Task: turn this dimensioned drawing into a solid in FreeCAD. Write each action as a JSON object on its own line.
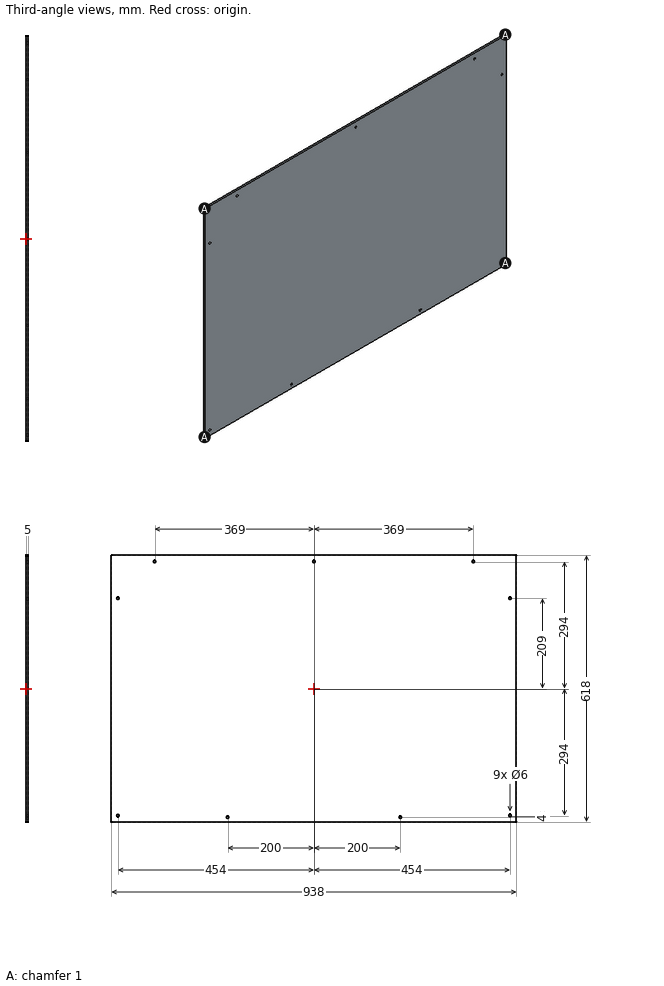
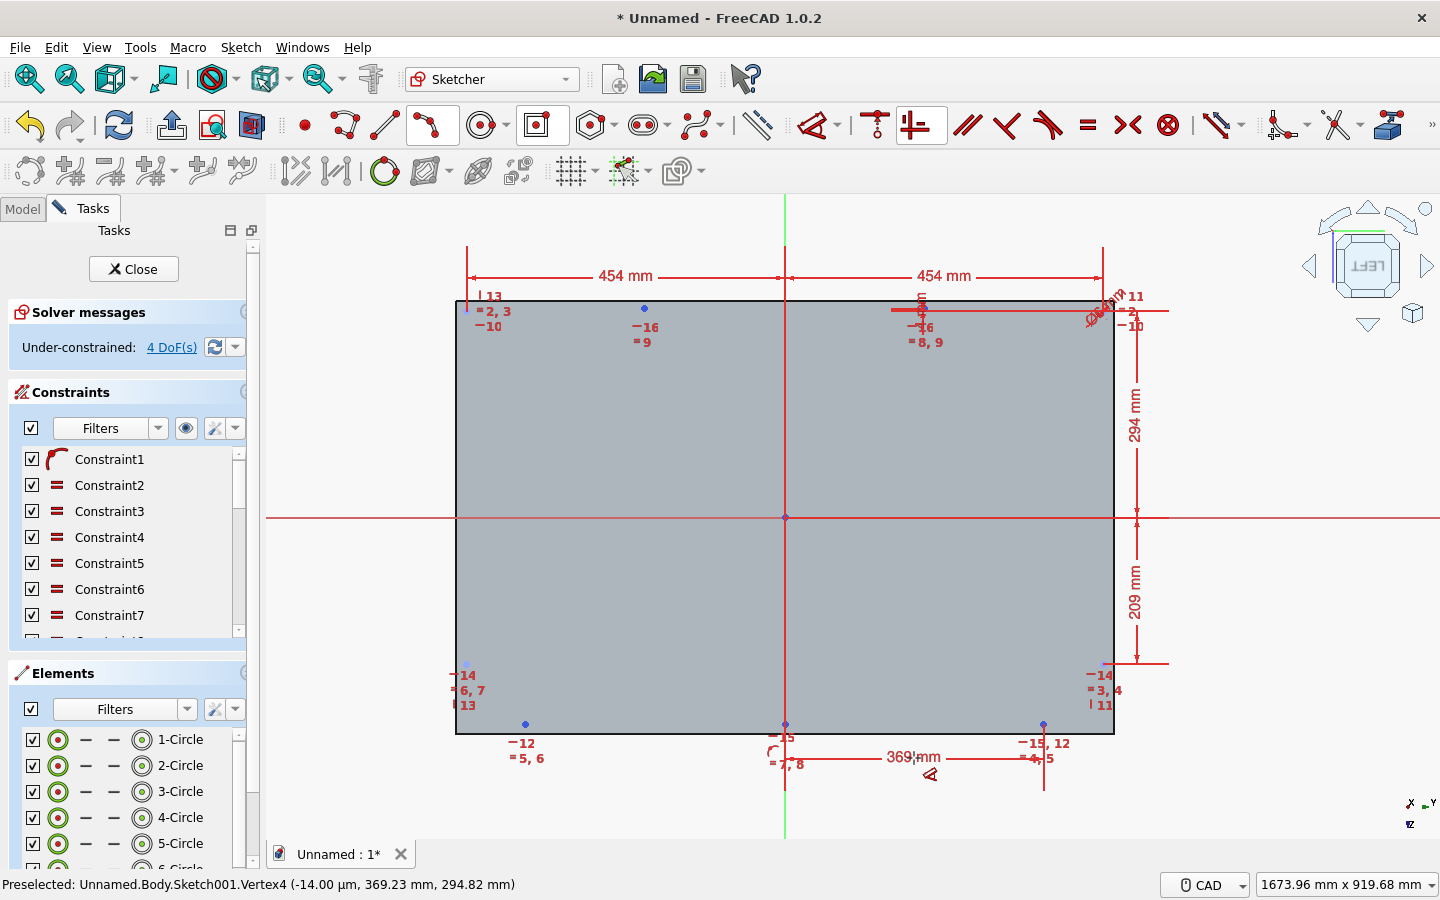
{"action": "left_click", "coordinate": [1044, 724]}
{"action": "left_click", "coordinate": [1078, 621]}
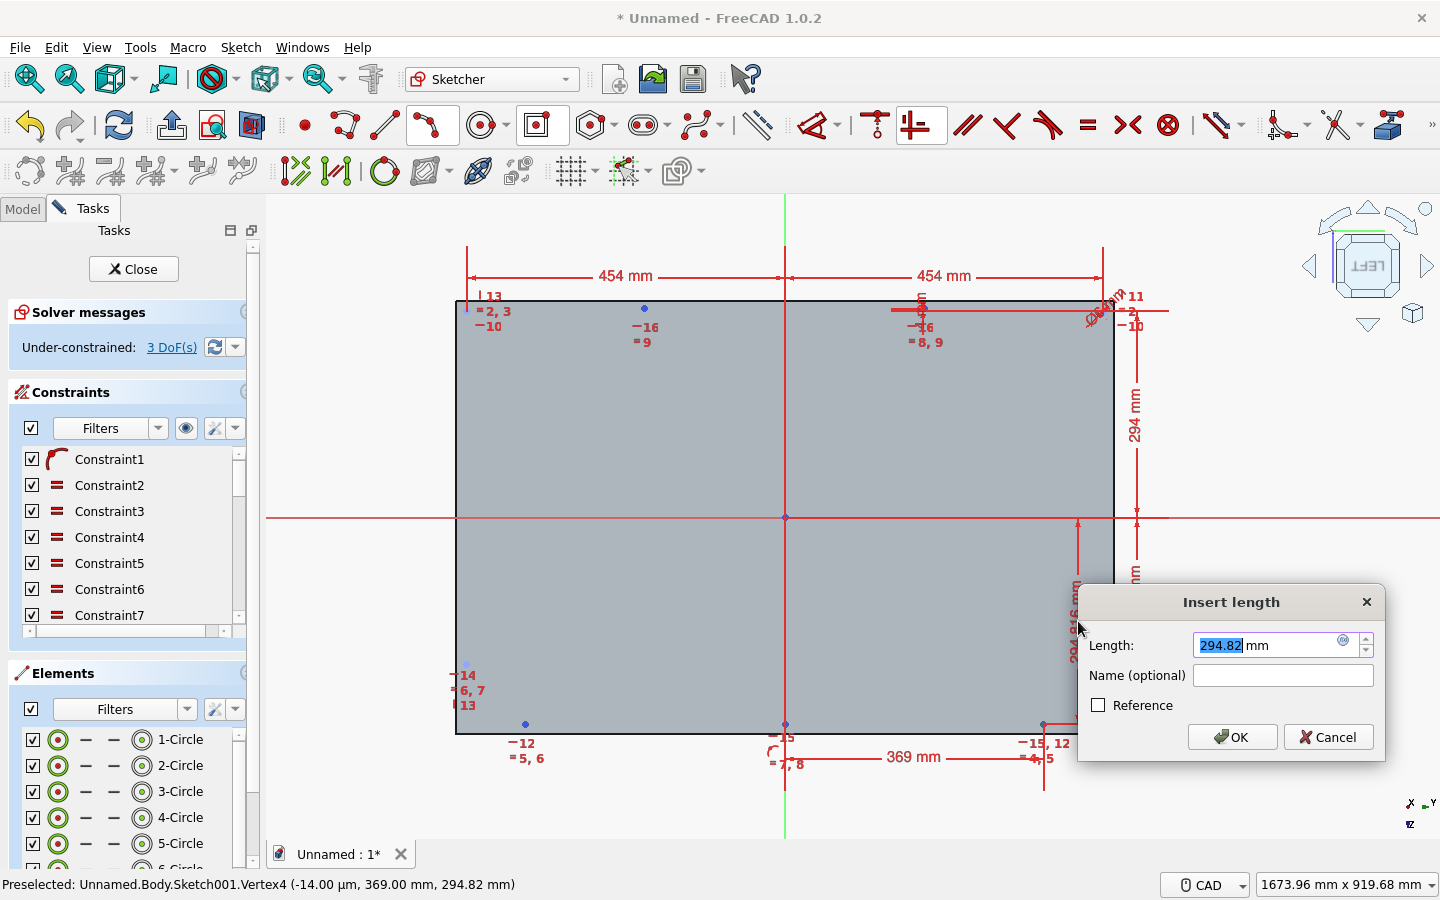
{"action": "type", "text": "294"}
{"action": "key", "text": "Return"}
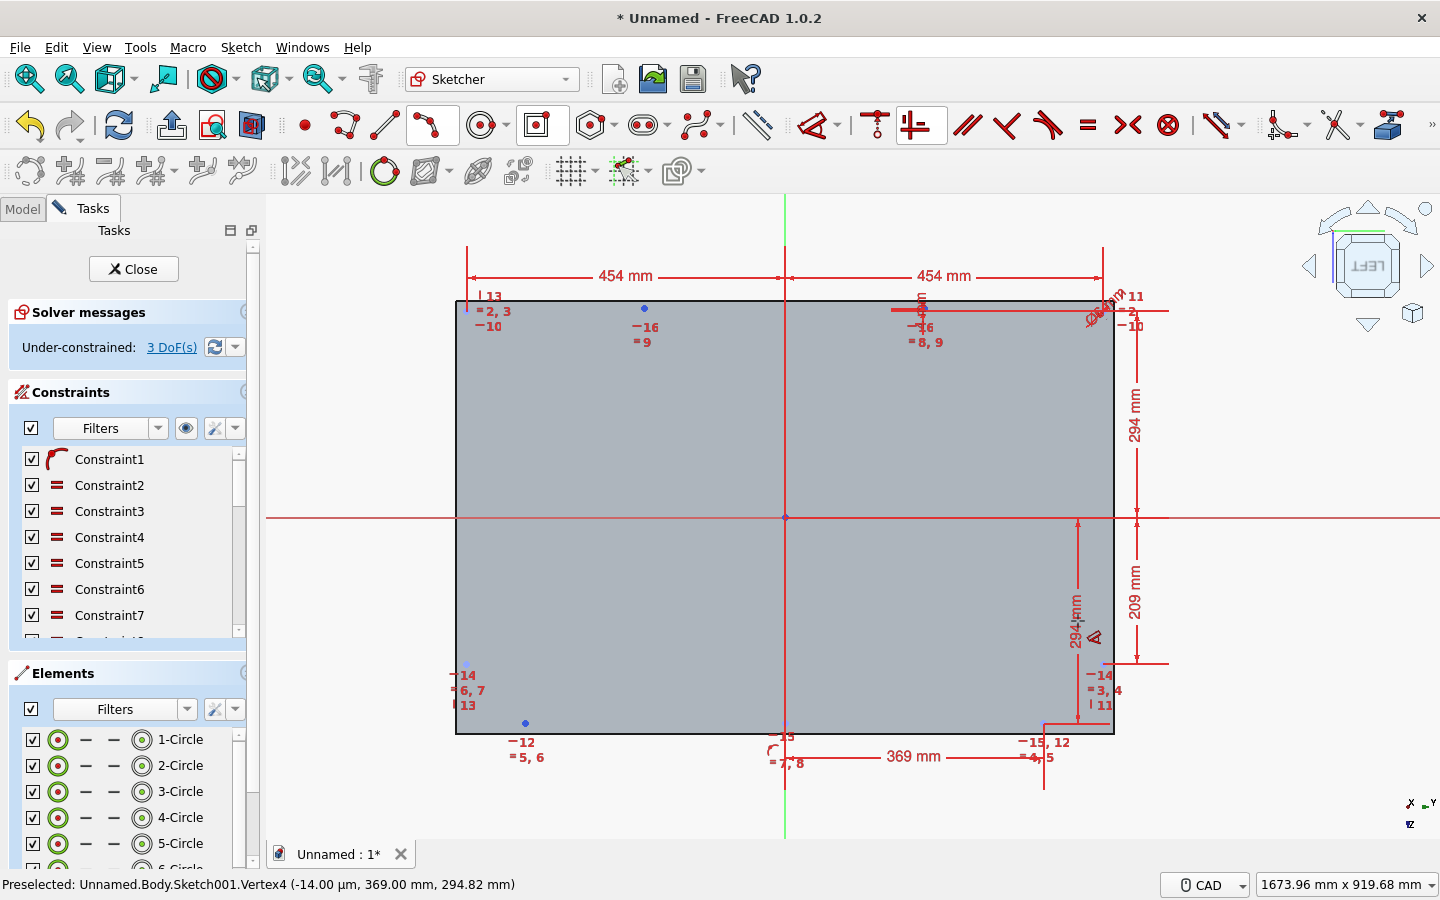
{"action": "left_click", "coordinate": [526, 724]}
{"action": "left_click", "coordinate": [655, 758]}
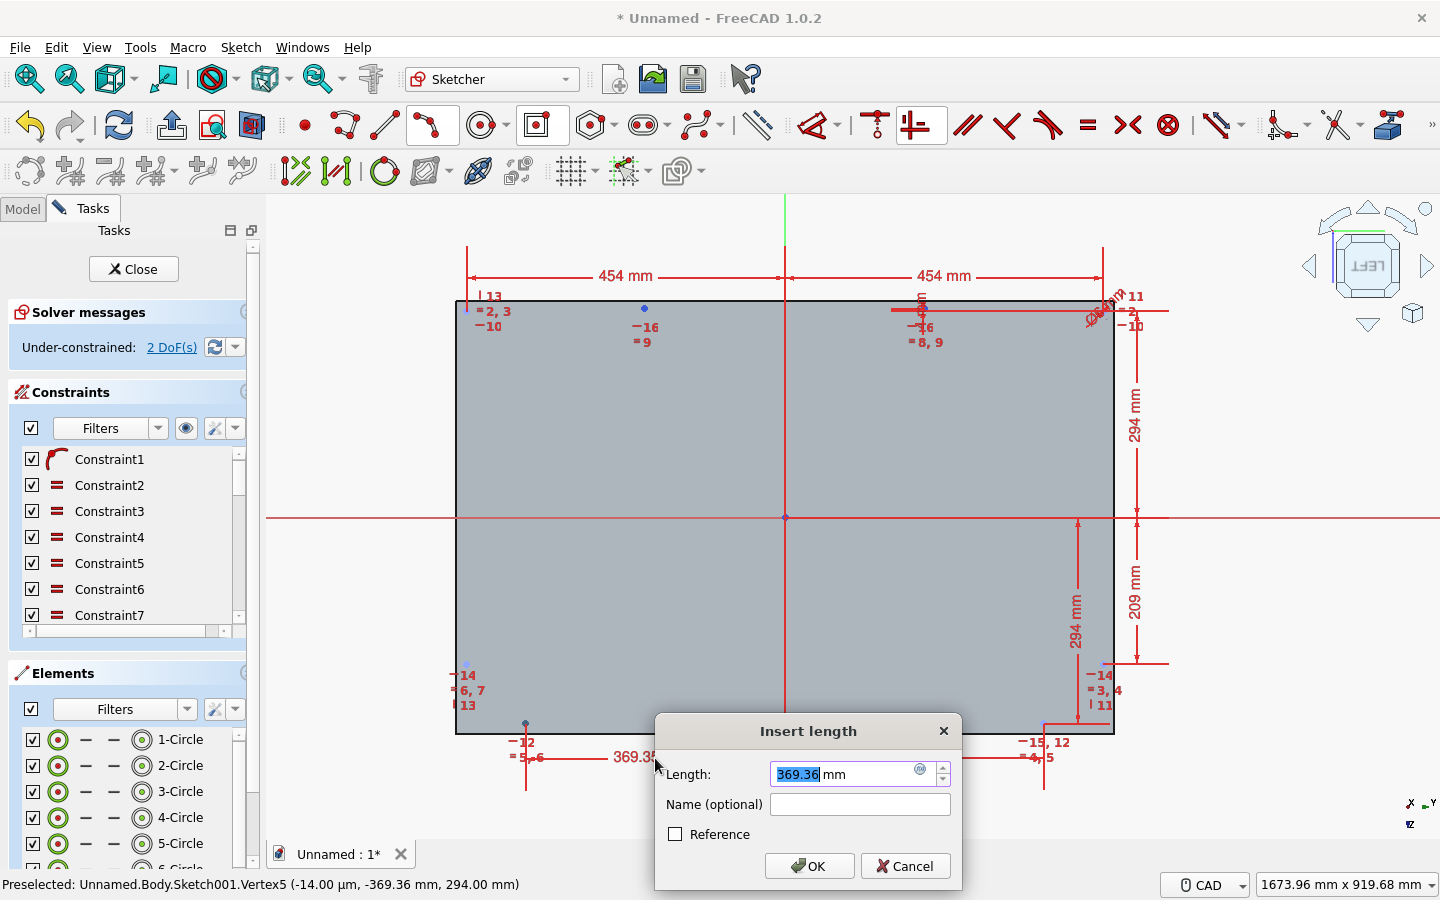
{"action": "type", "text": "369"}
{"action": "key", "text": "Return"}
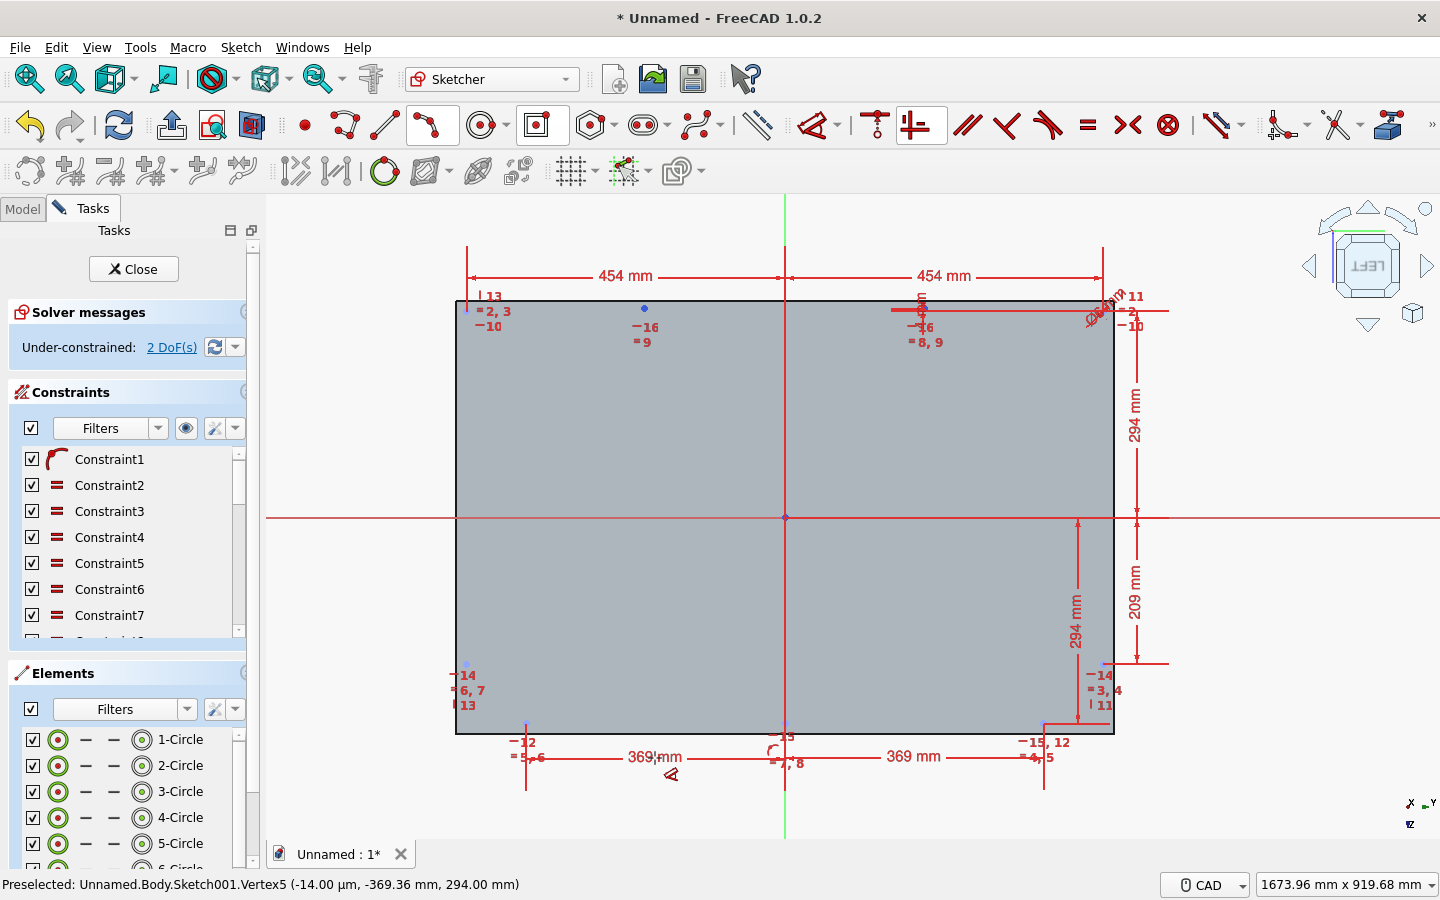
{"action": "left_click", "coordinate": [925, 309]}
{"action": "left_click", "coordinate": [855, 275]}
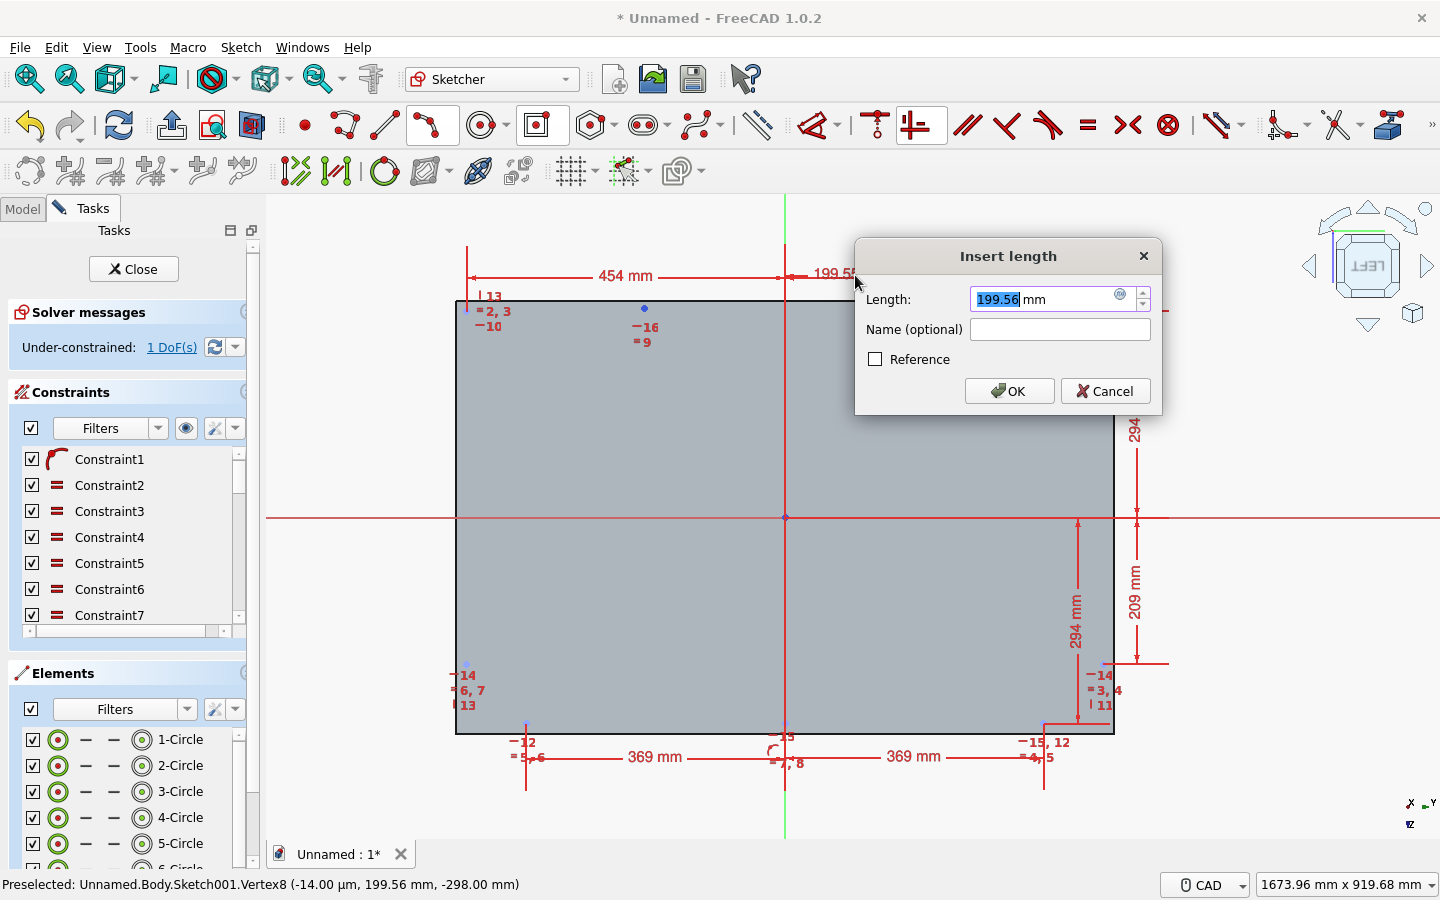
{"action": "type", "text": "200"}
{"action": "key", "text": "Return"}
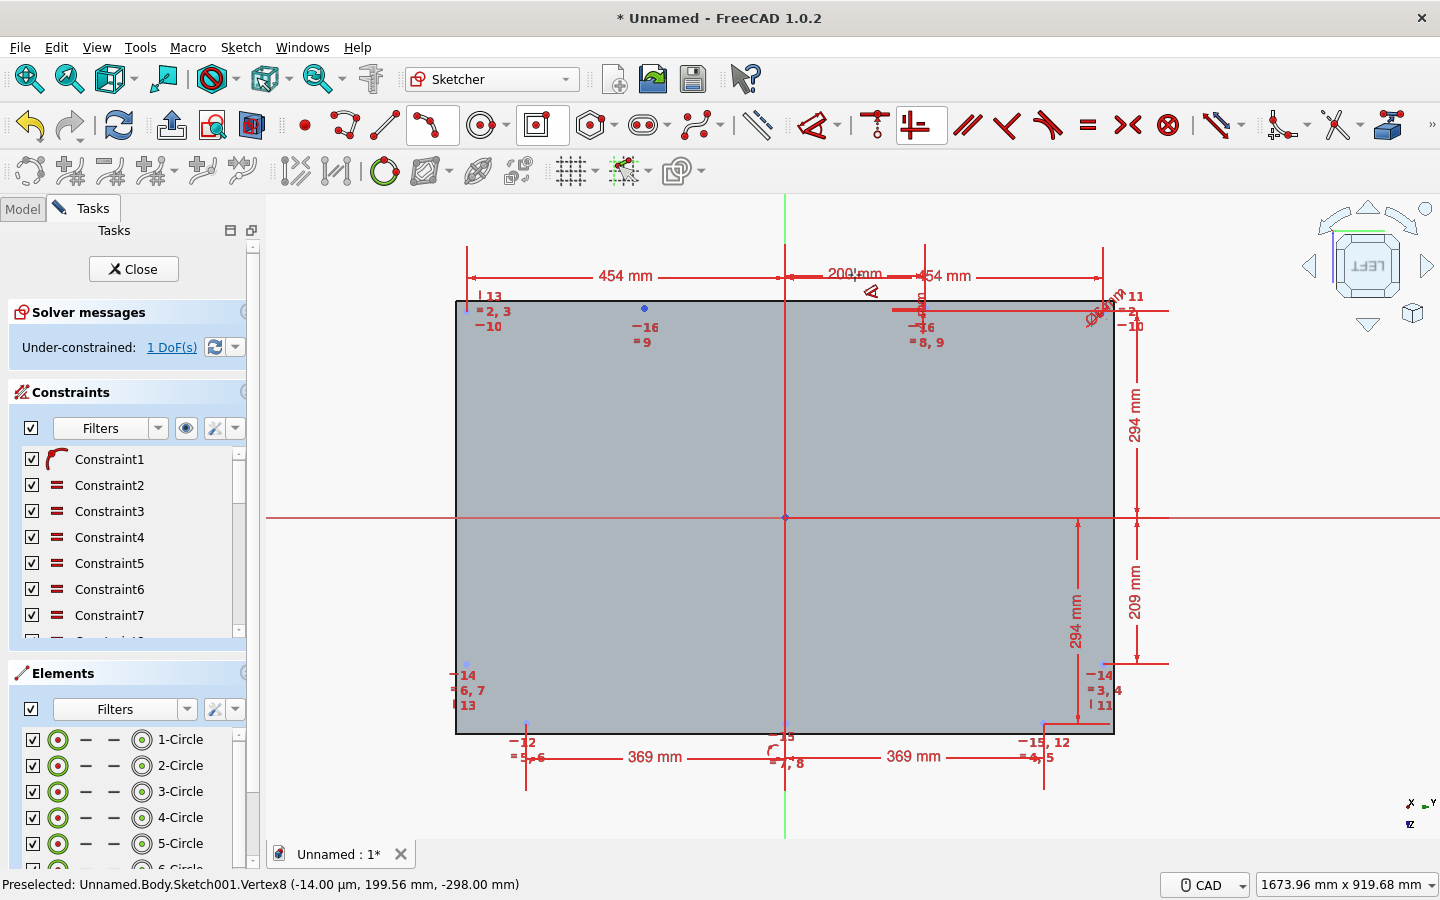
{"action": "left_click", "coordinate": [645, 309]}
{"action": "left_click", "coordinate": [715, 275]}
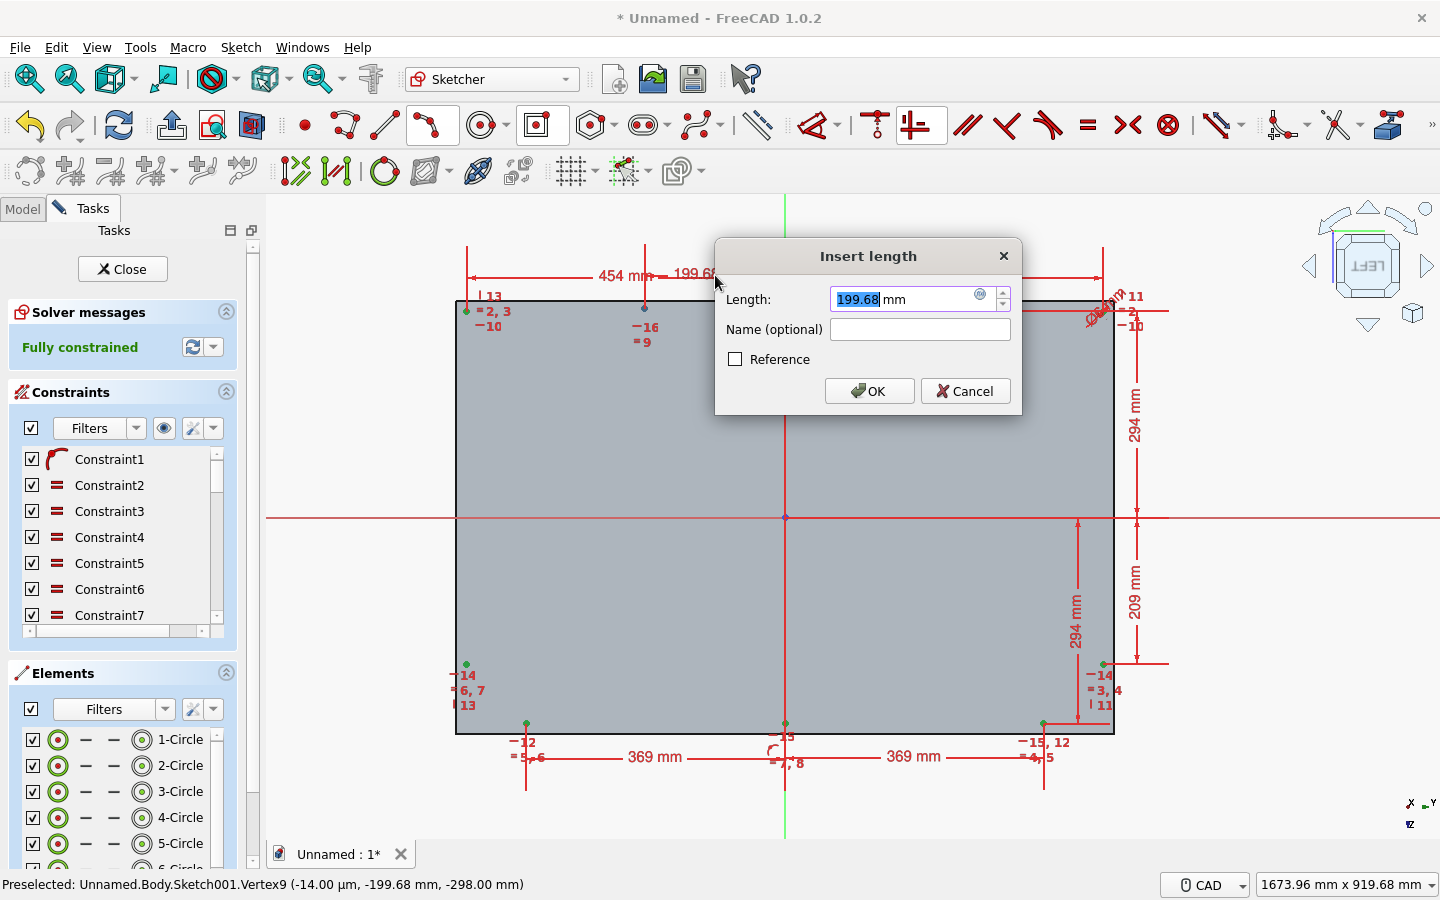
{"action": "type", "text": "200"}
{"action": "key", "text": "Return"}
{"action": "key", "text": "Escape"}